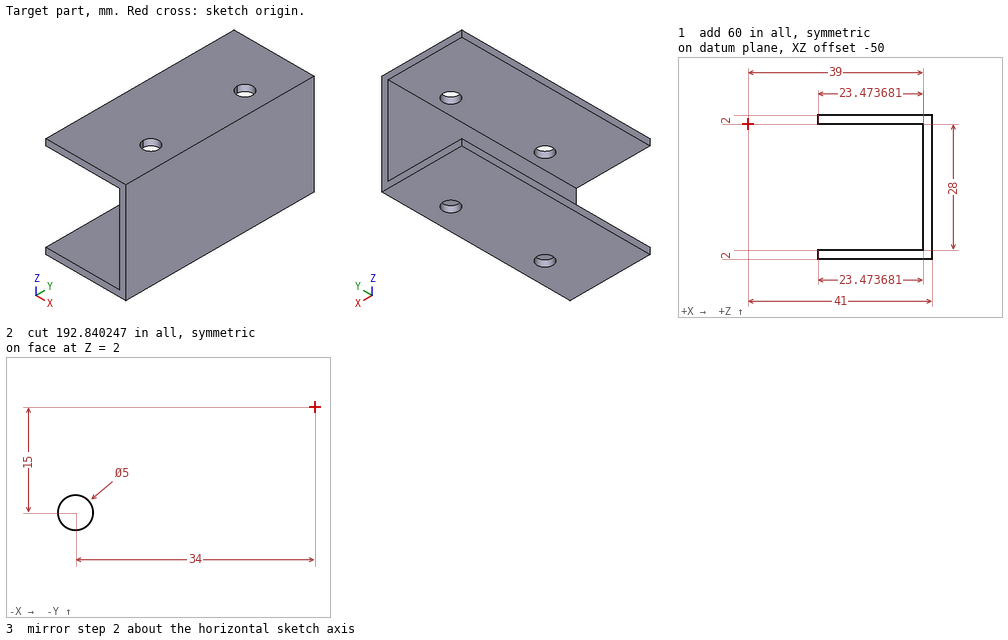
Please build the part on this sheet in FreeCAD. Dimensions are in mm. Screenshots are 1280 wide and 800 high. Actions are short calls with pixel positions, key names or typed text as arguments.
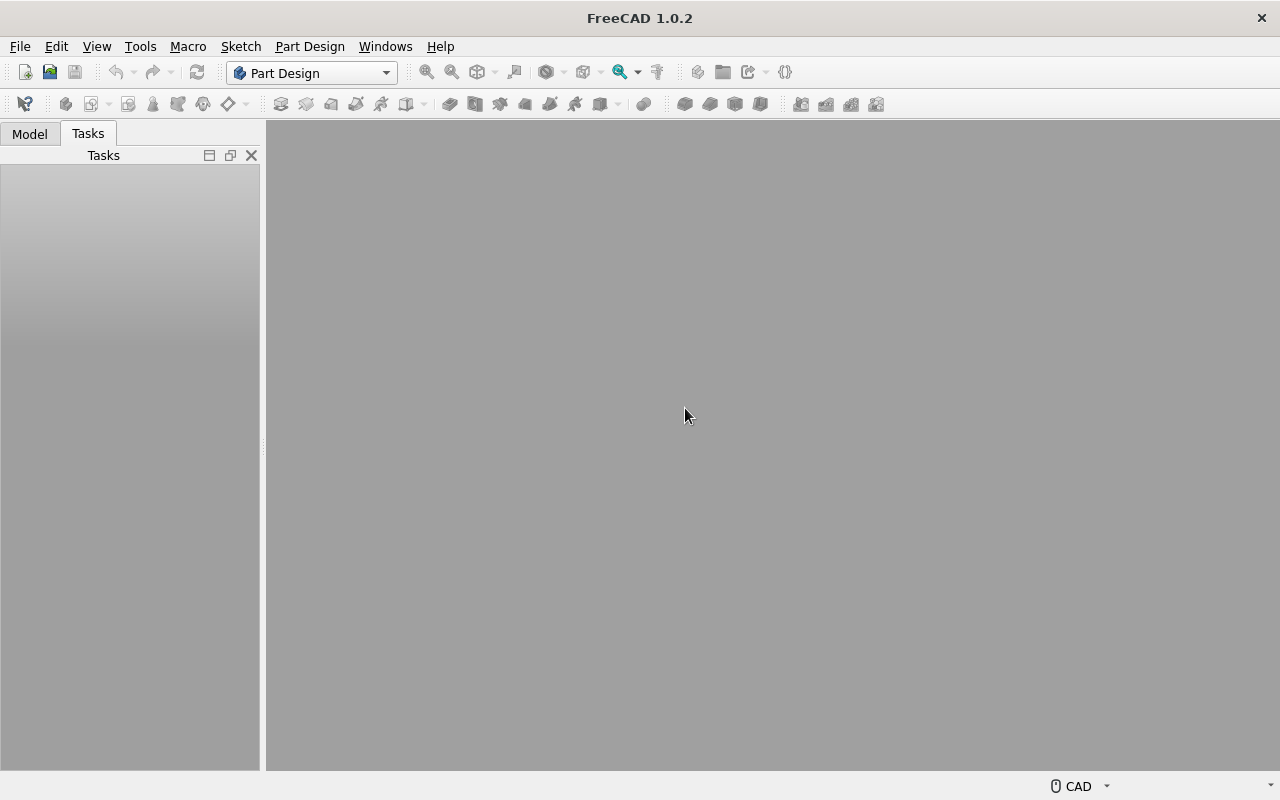
click(25, 72)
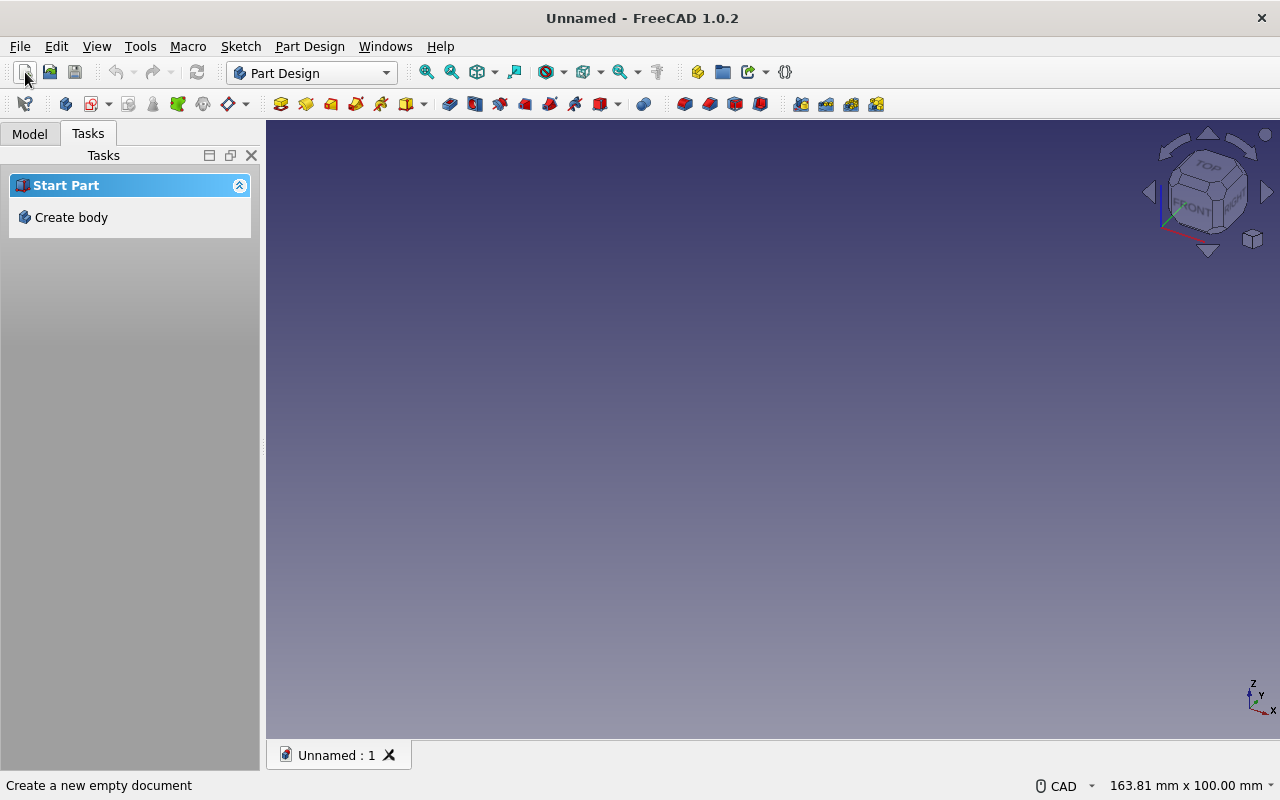
click(66, 104)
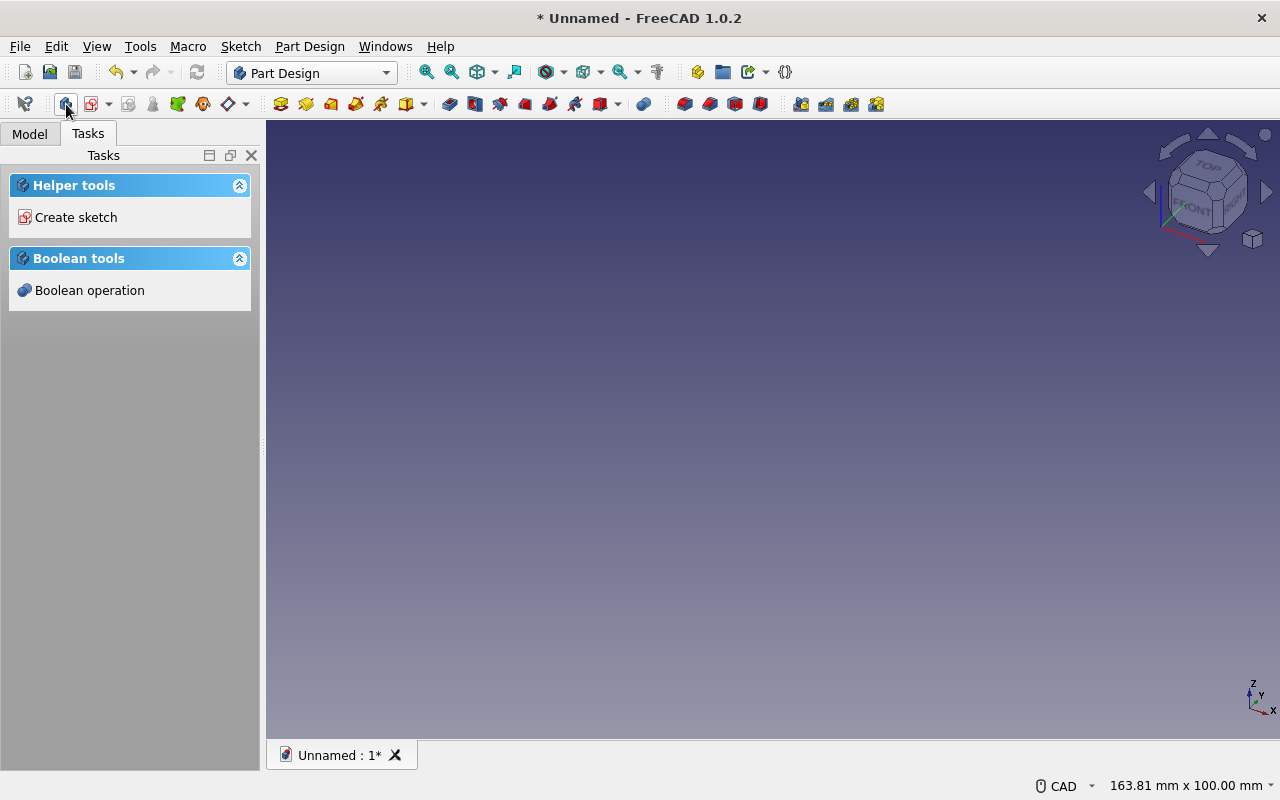
click(30, 134)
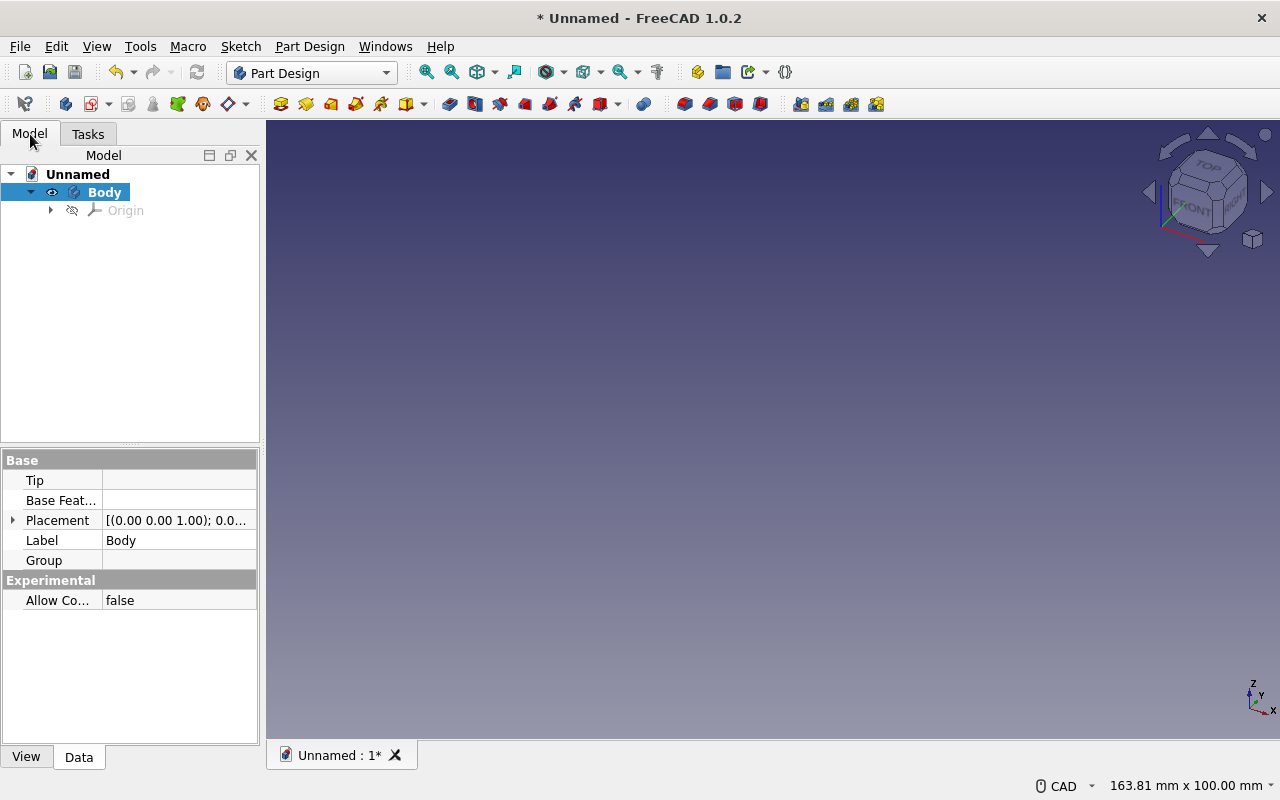
click(51, 210)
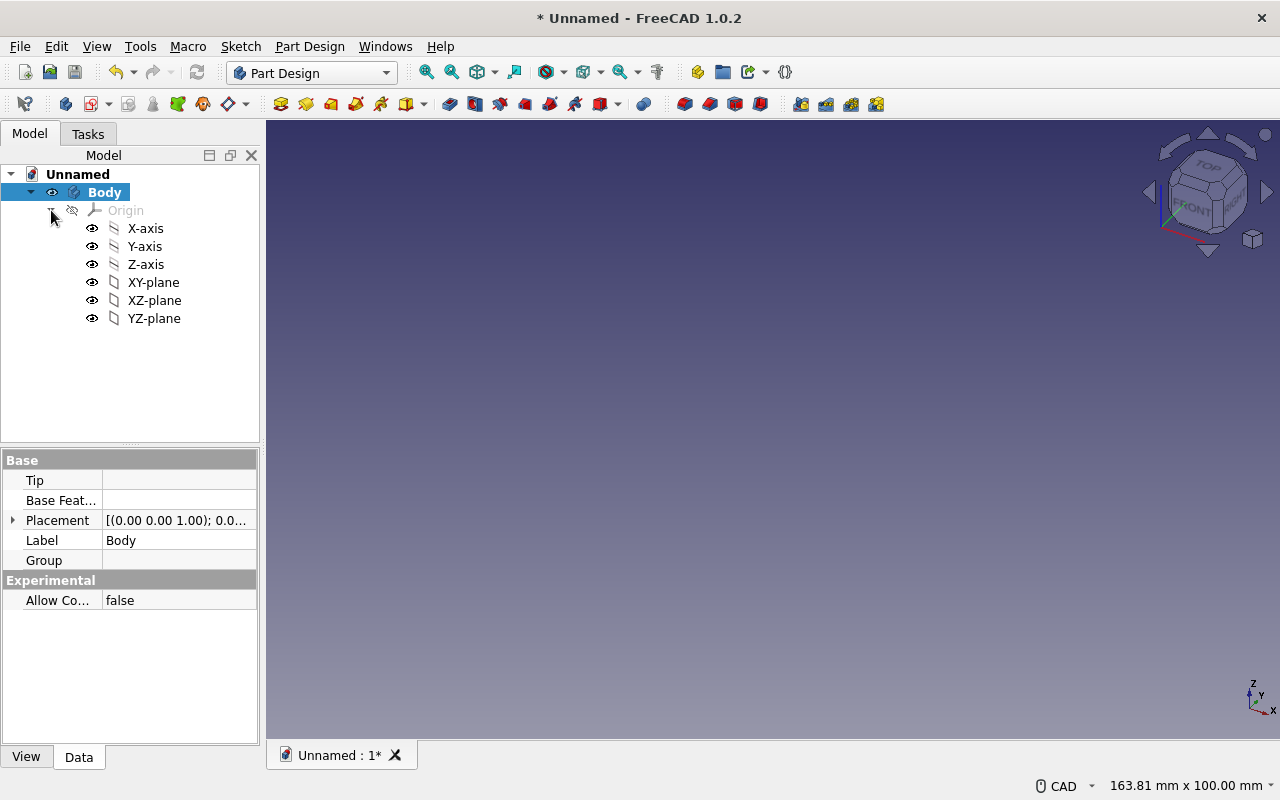
click(137, 300)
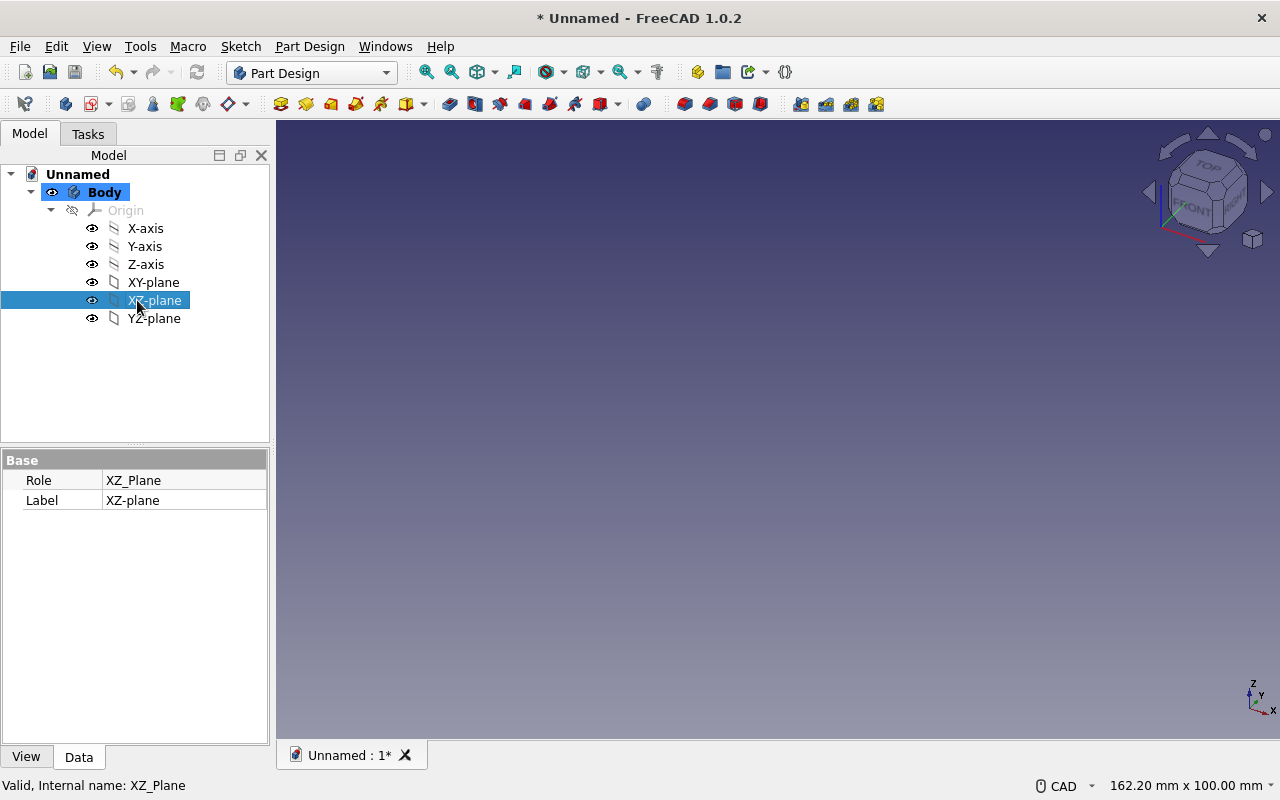
click(228, 104)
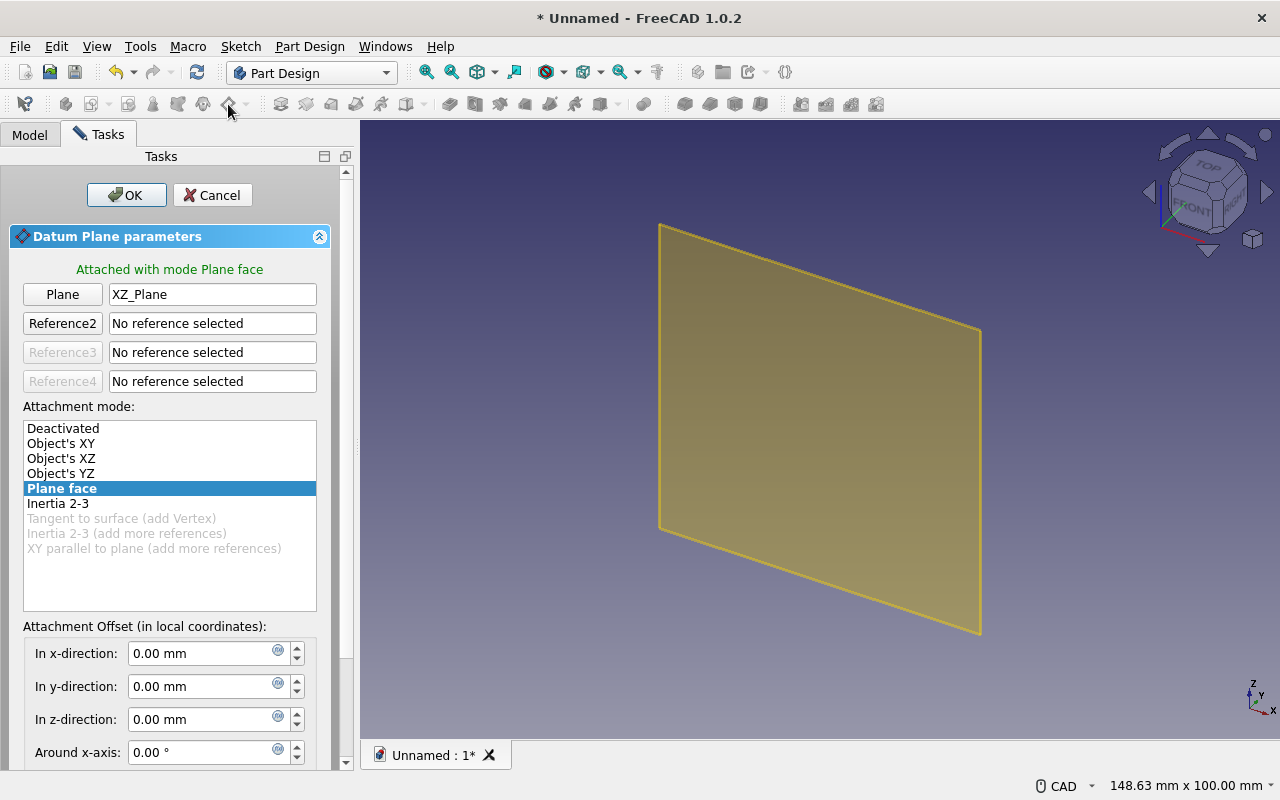
triple_click(210, 720)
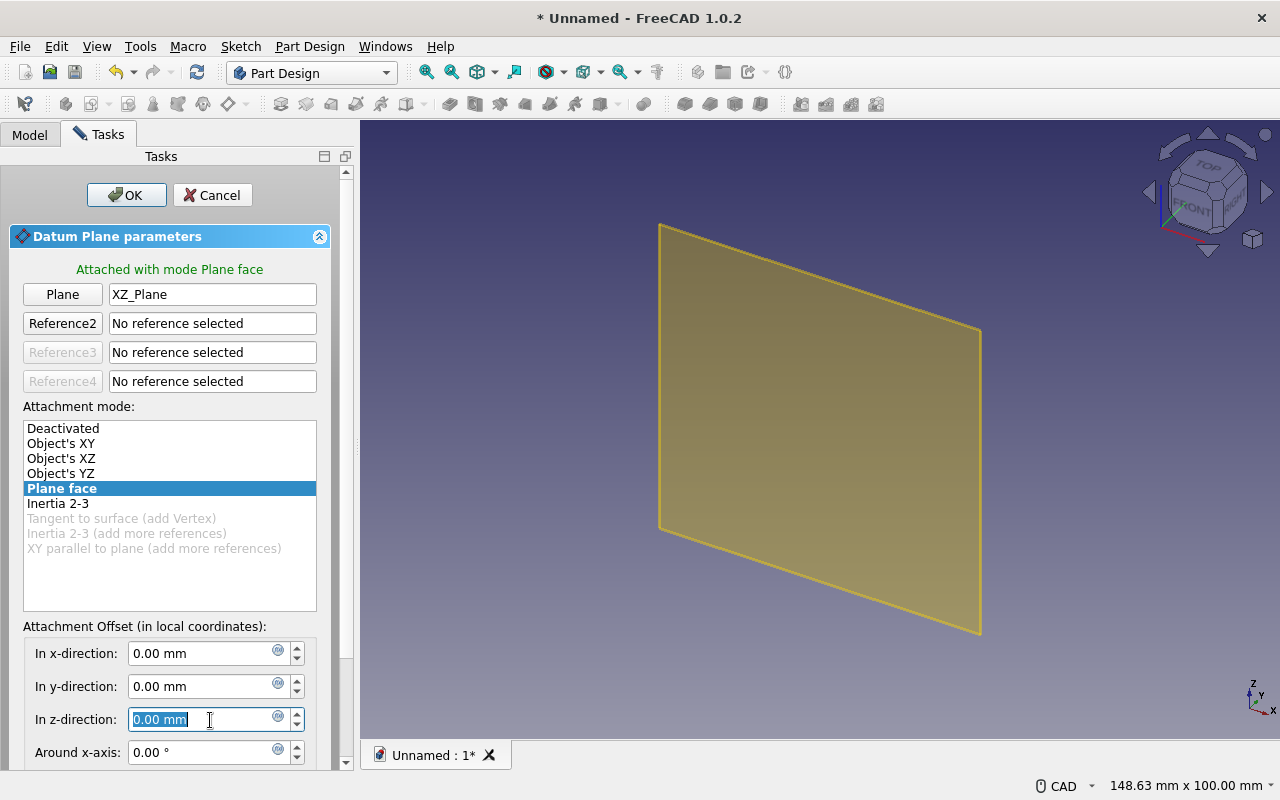
text(-50)
key(Tab)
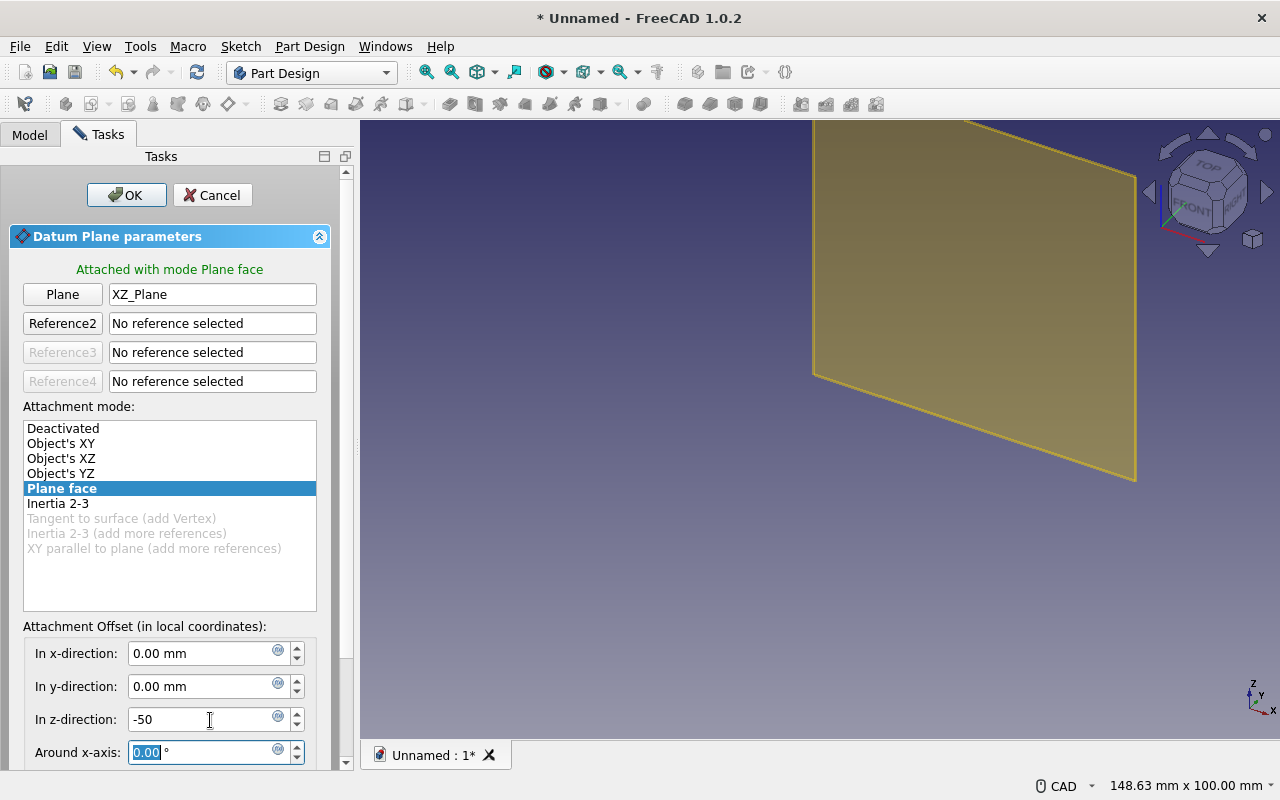
click(127, 195)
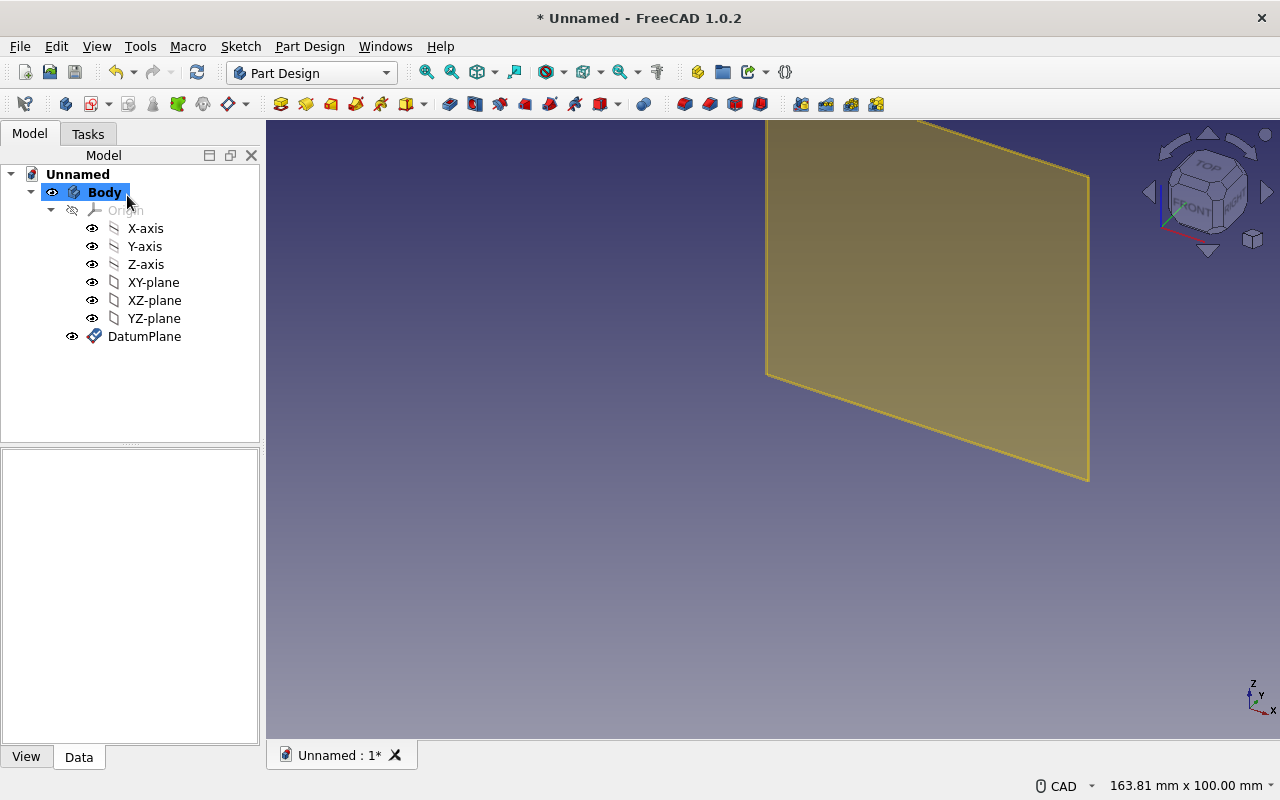
click(117, 336)